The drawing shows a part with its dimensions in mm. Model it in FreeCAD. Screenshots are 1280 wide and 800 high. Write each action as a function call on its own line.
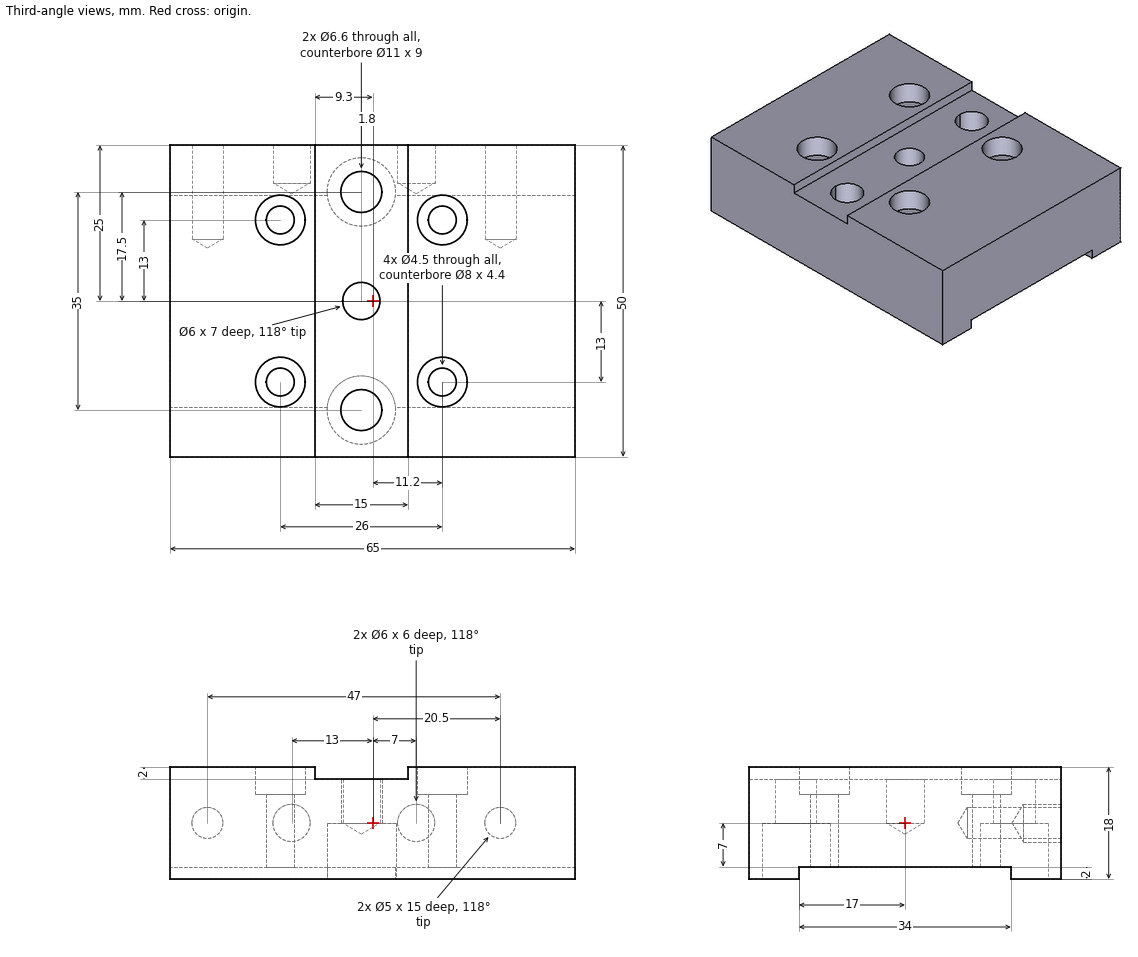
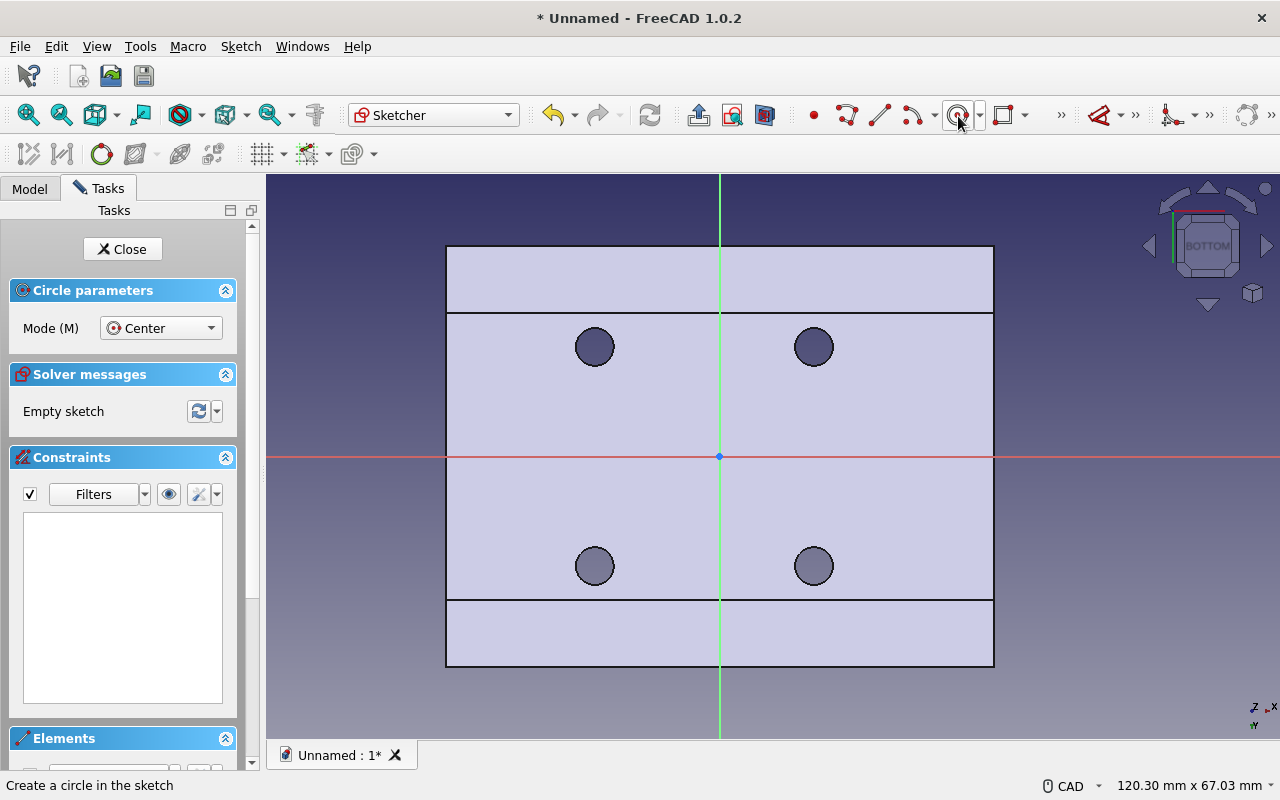
click(704, 604)
move(685, 584)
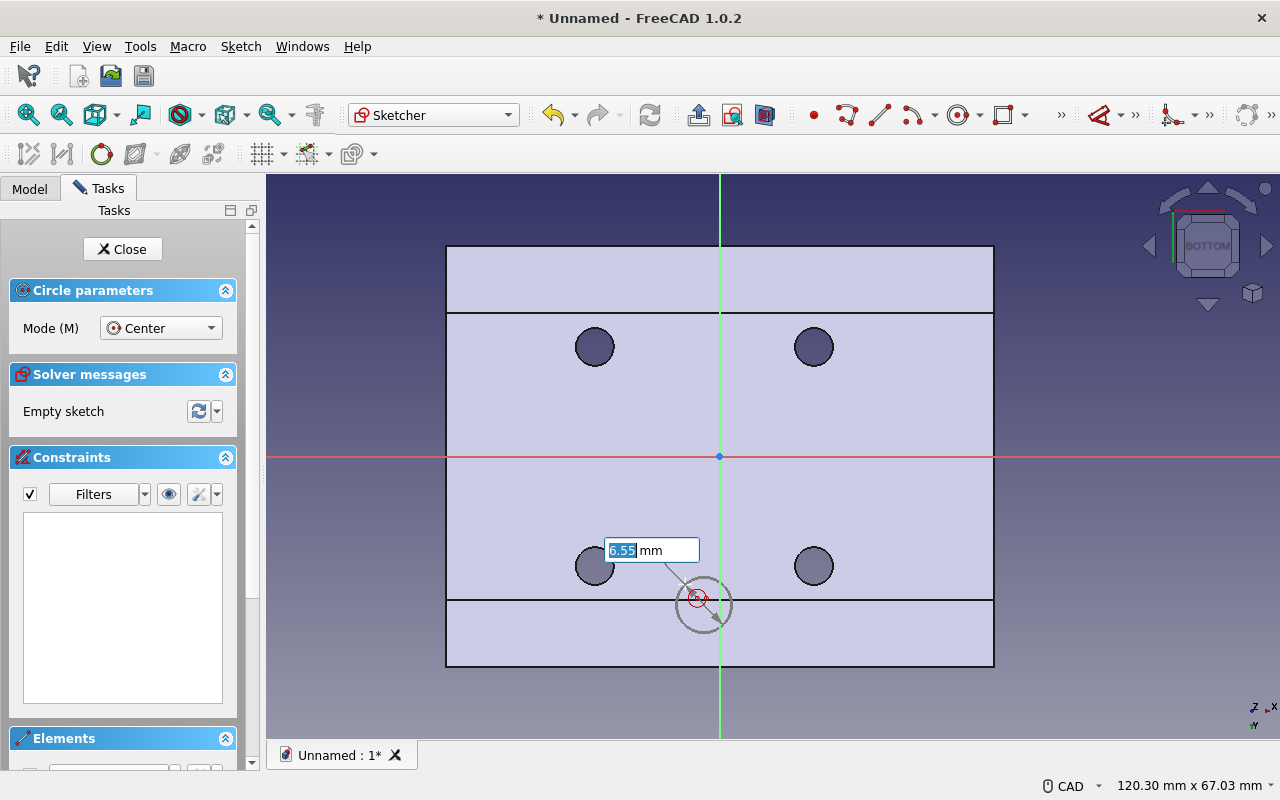
text(6.6)
key(Return)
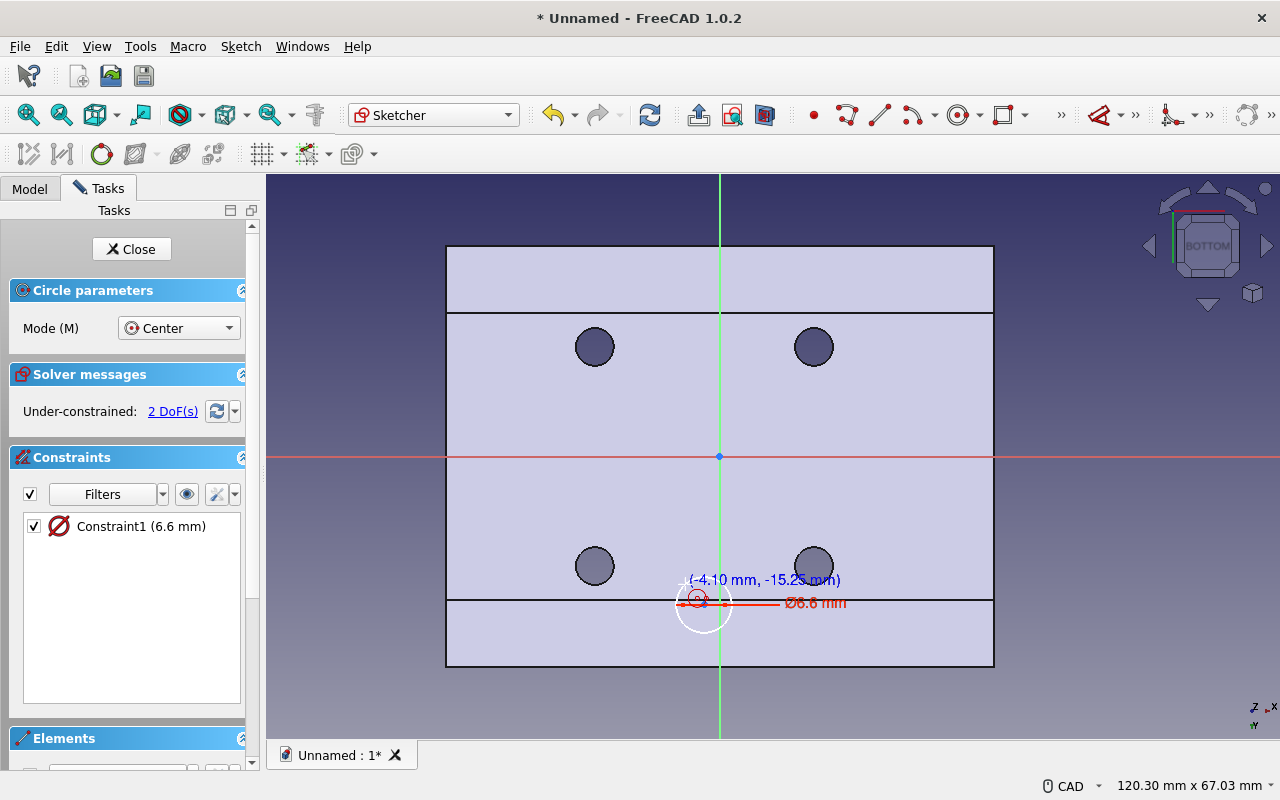
click(704, 309)
move(685, 289)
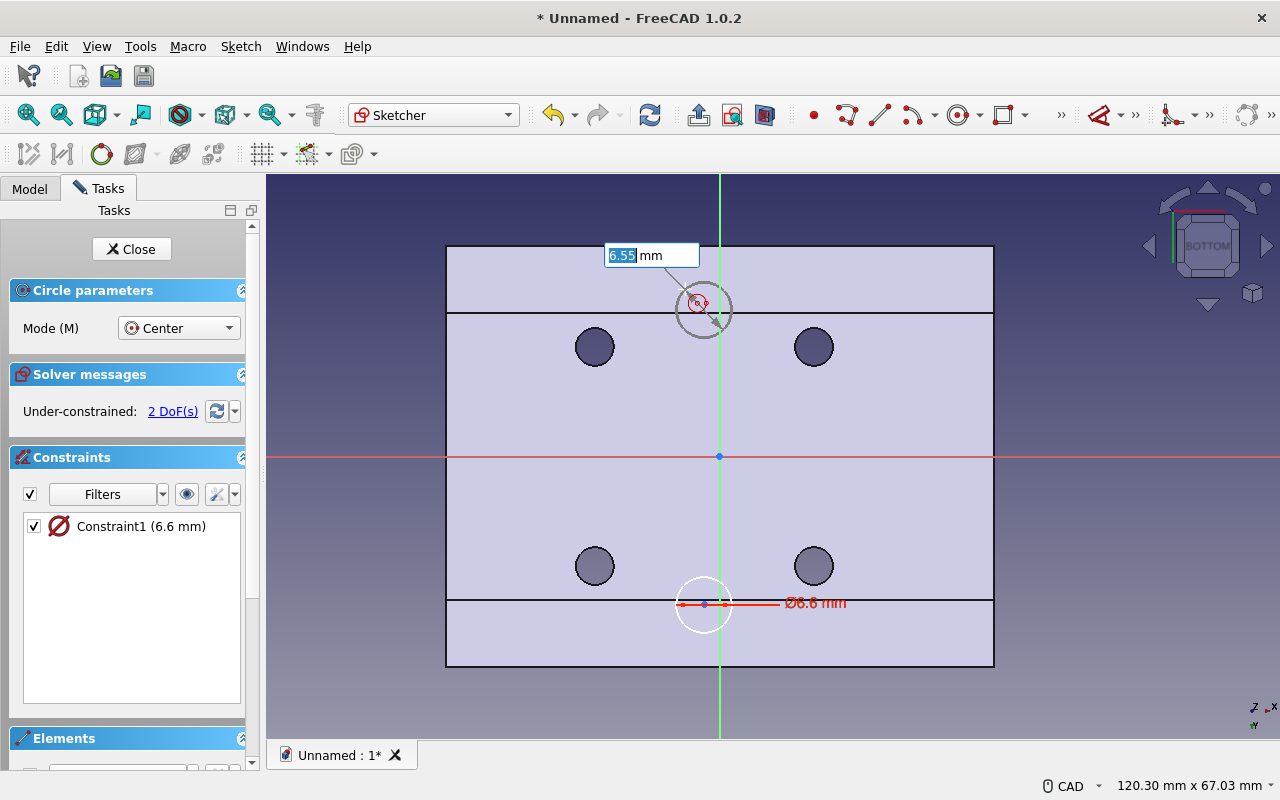
text(6.6)
key(Return)
key(Escape)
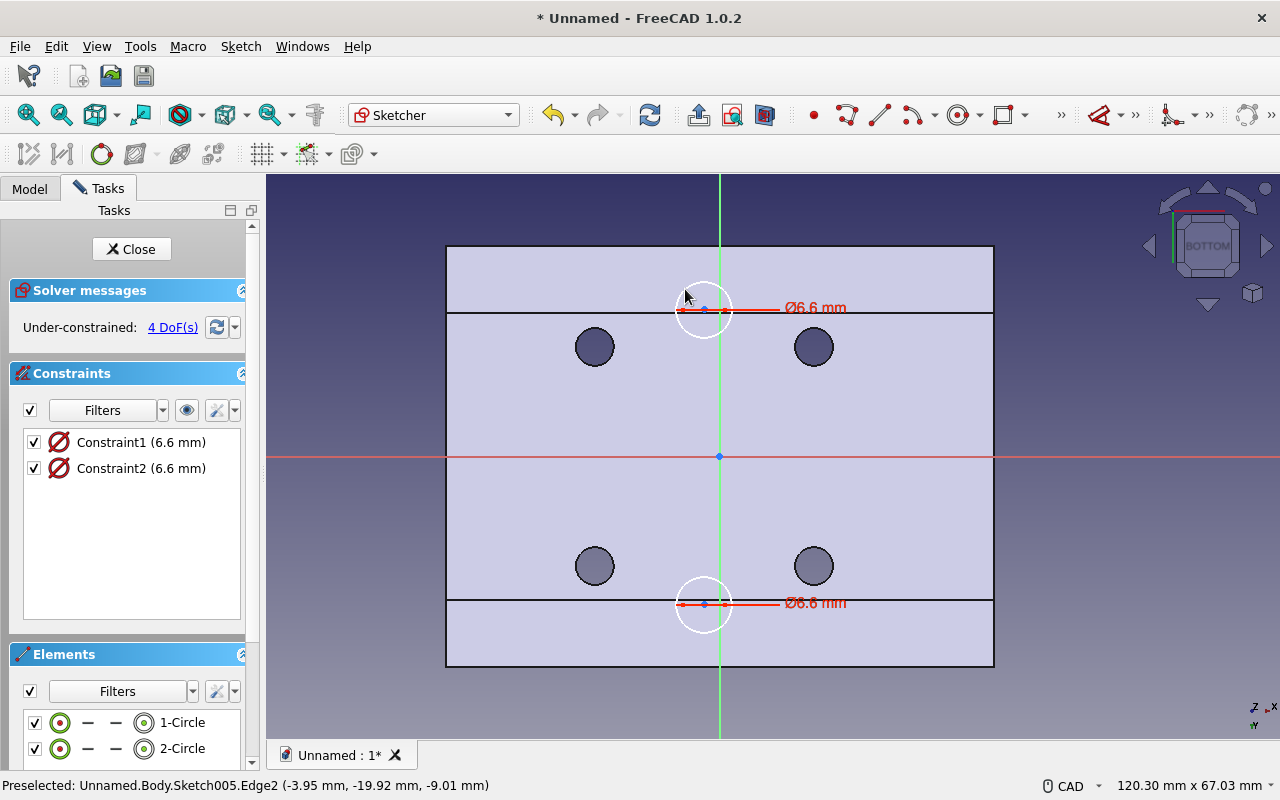
click(704, 605)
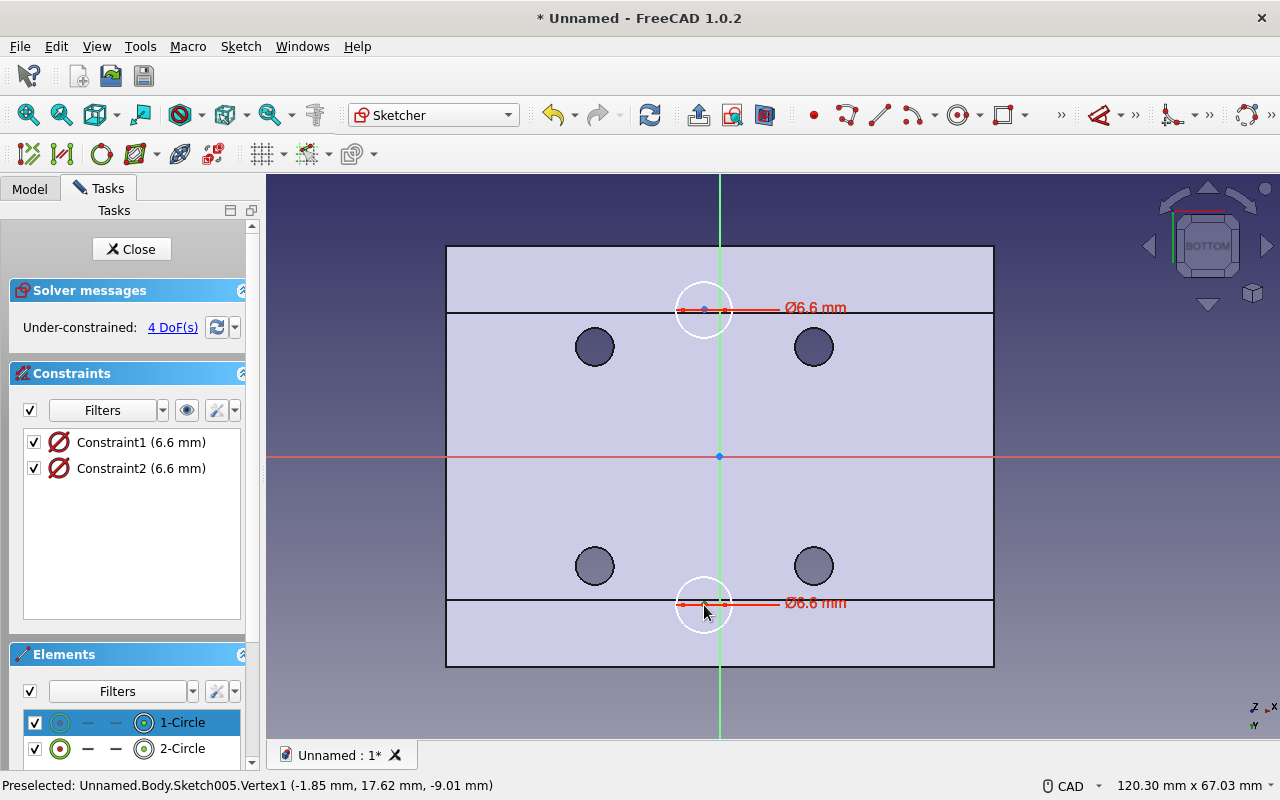
click(704, 310)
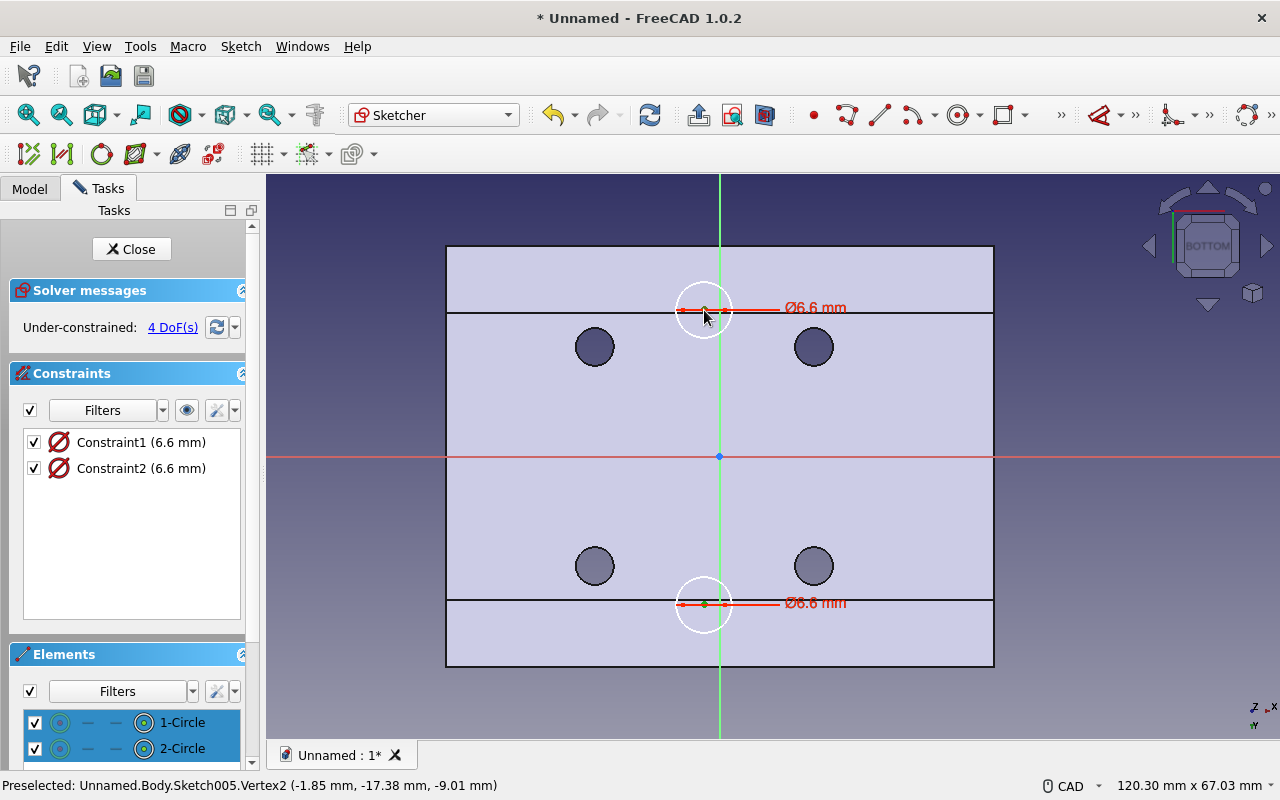
key(v)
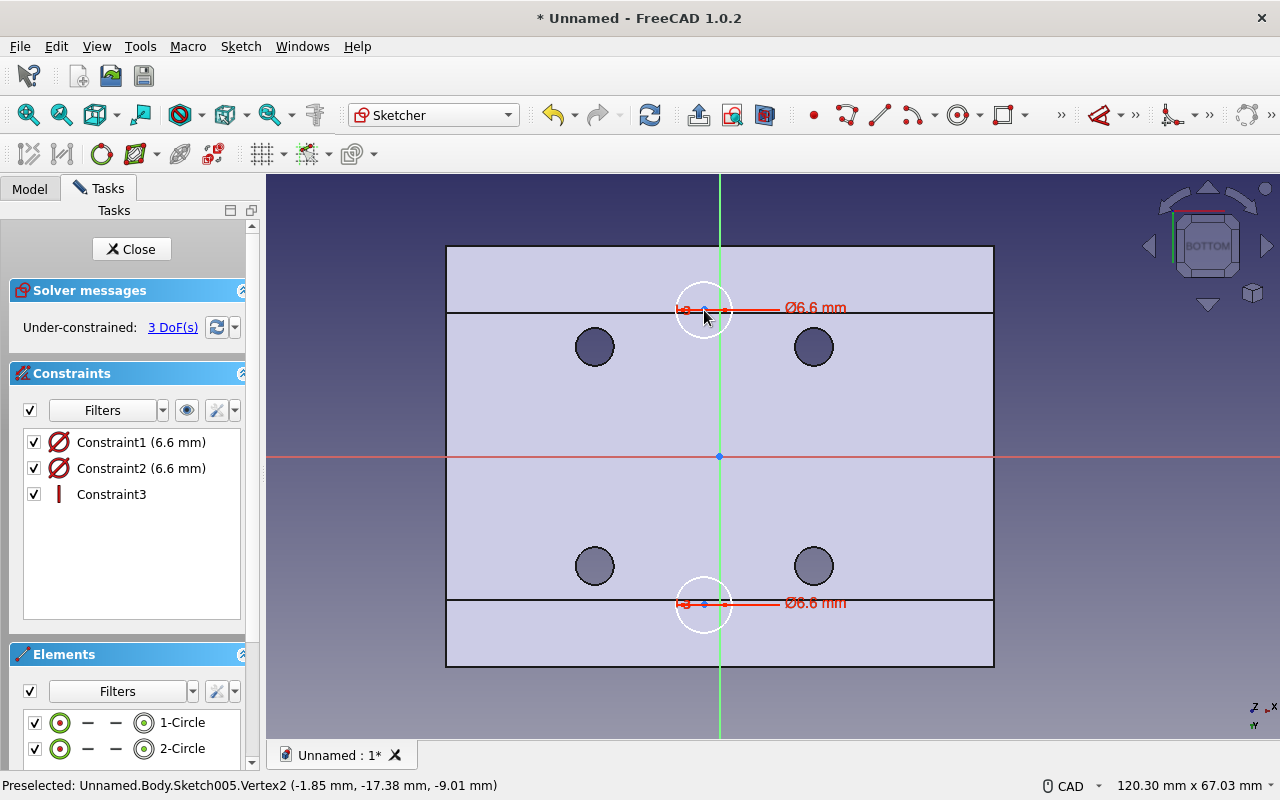
key(d)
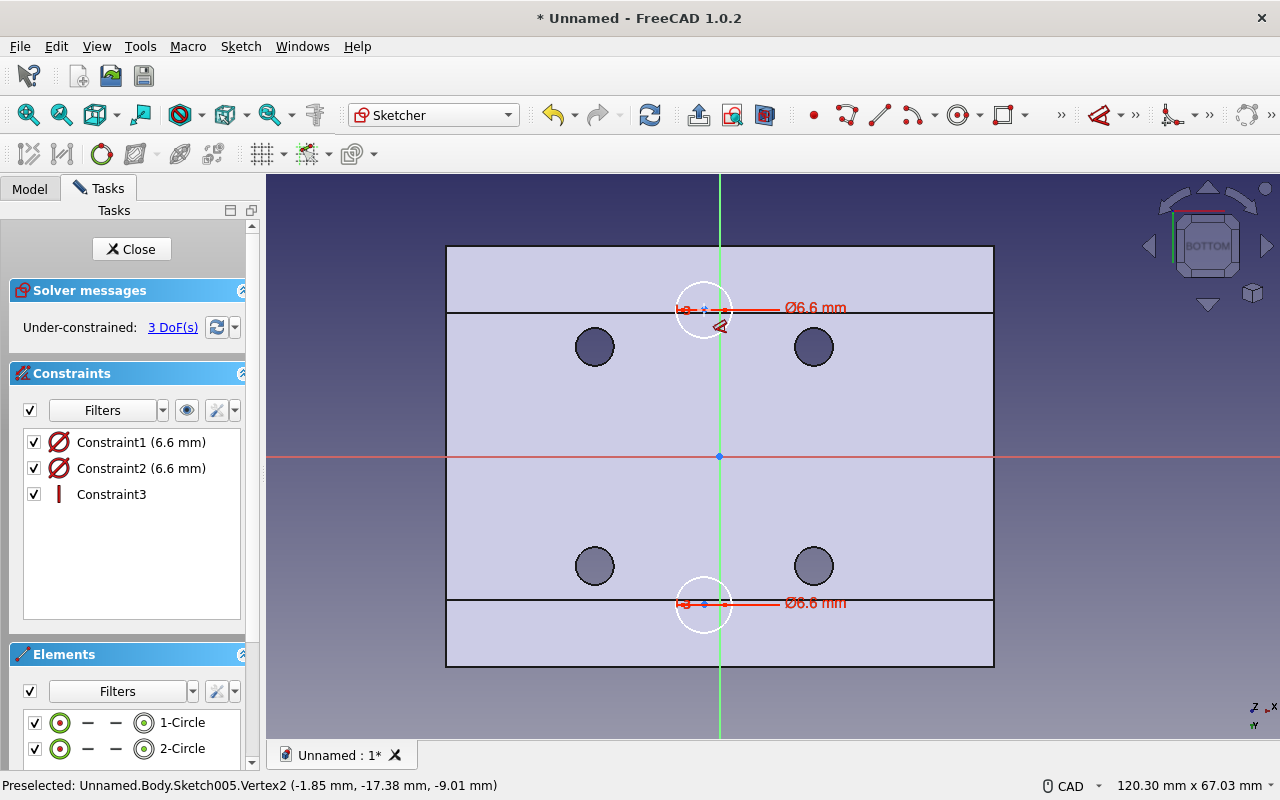
scroll(704, 605, up, 5)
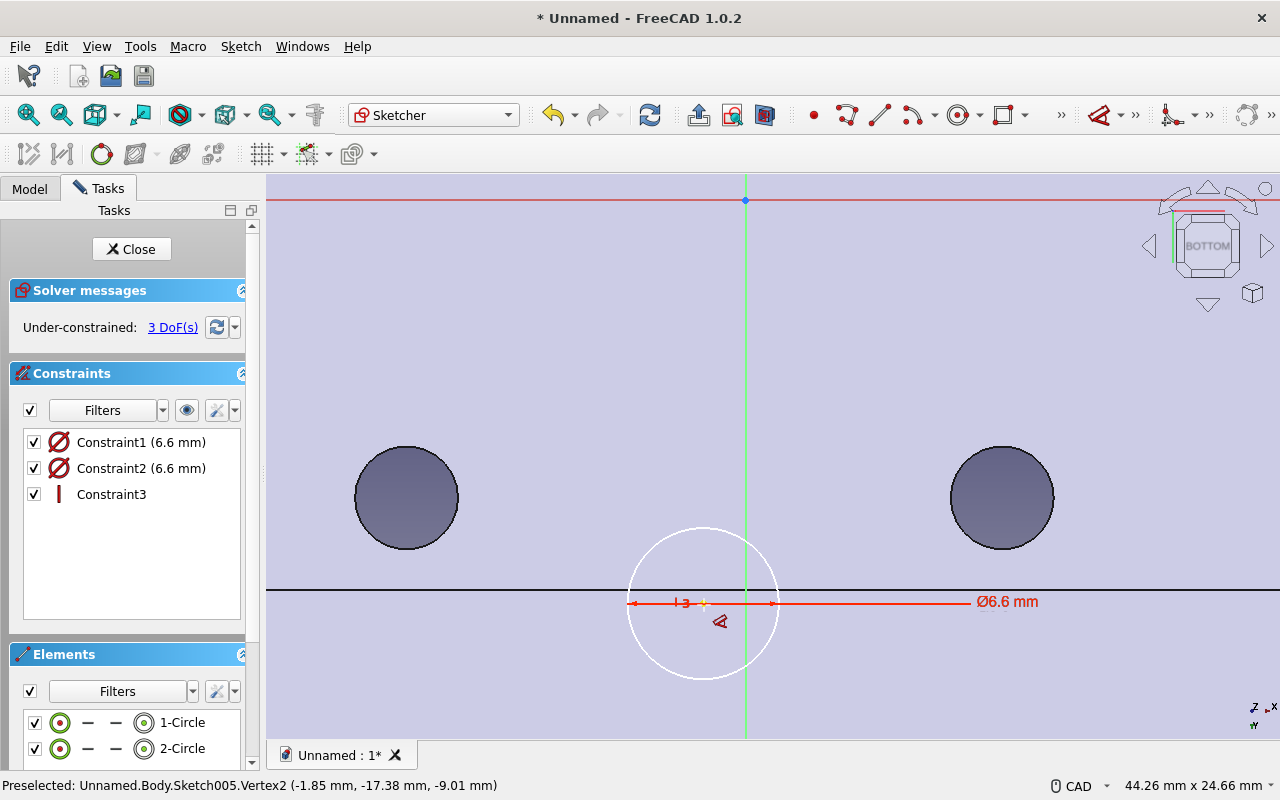
click(703, 604)
click(724, 638)